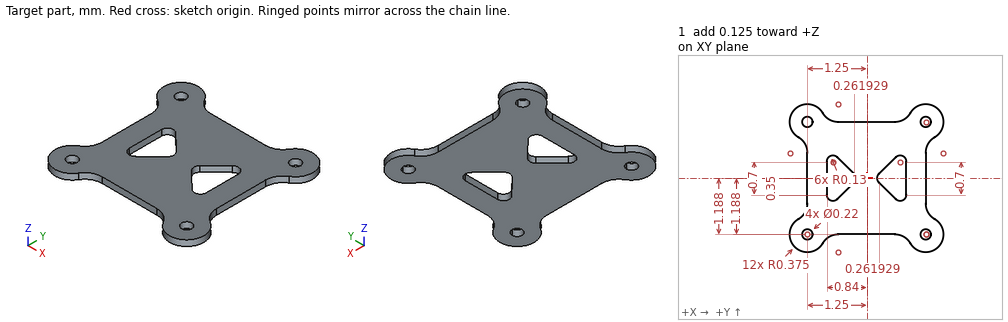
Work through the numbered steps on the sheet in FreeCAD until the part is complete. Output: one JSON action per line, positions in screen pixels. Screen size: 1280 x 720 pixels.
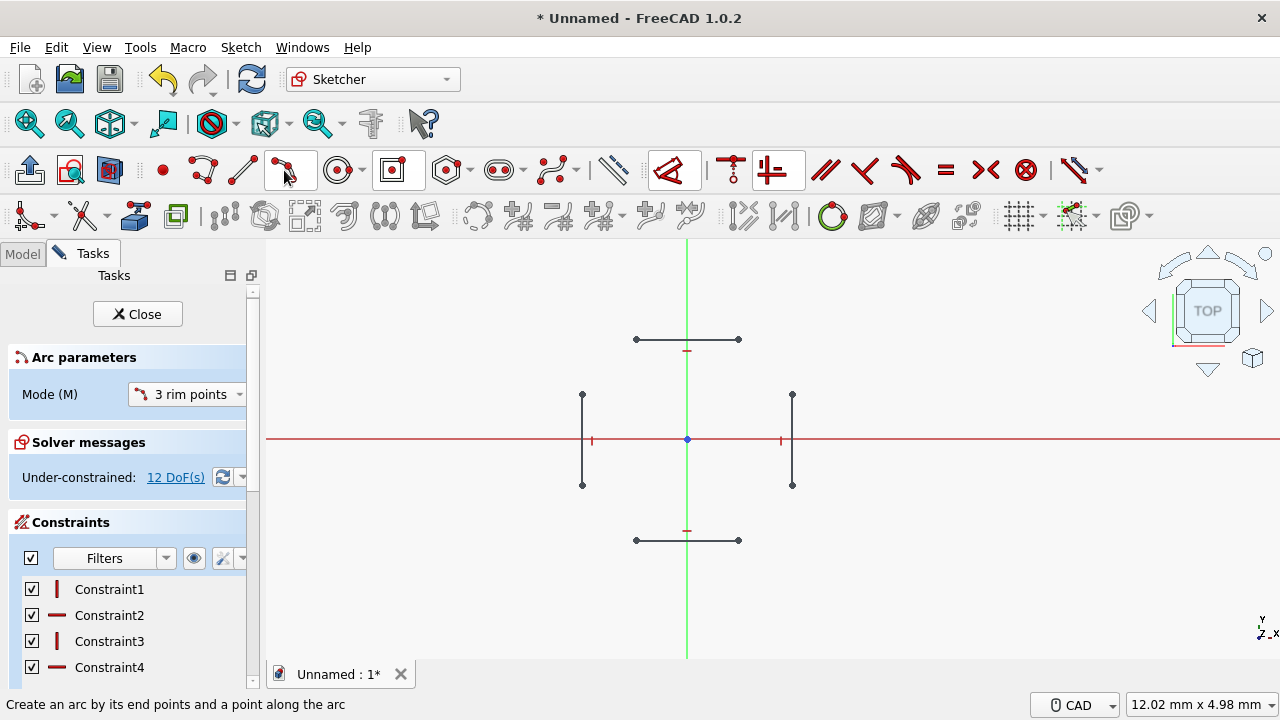
{"action": "left_click", "coordinate": [582, 486]}
{"action": "left_click", "coordinate": [566, 512]}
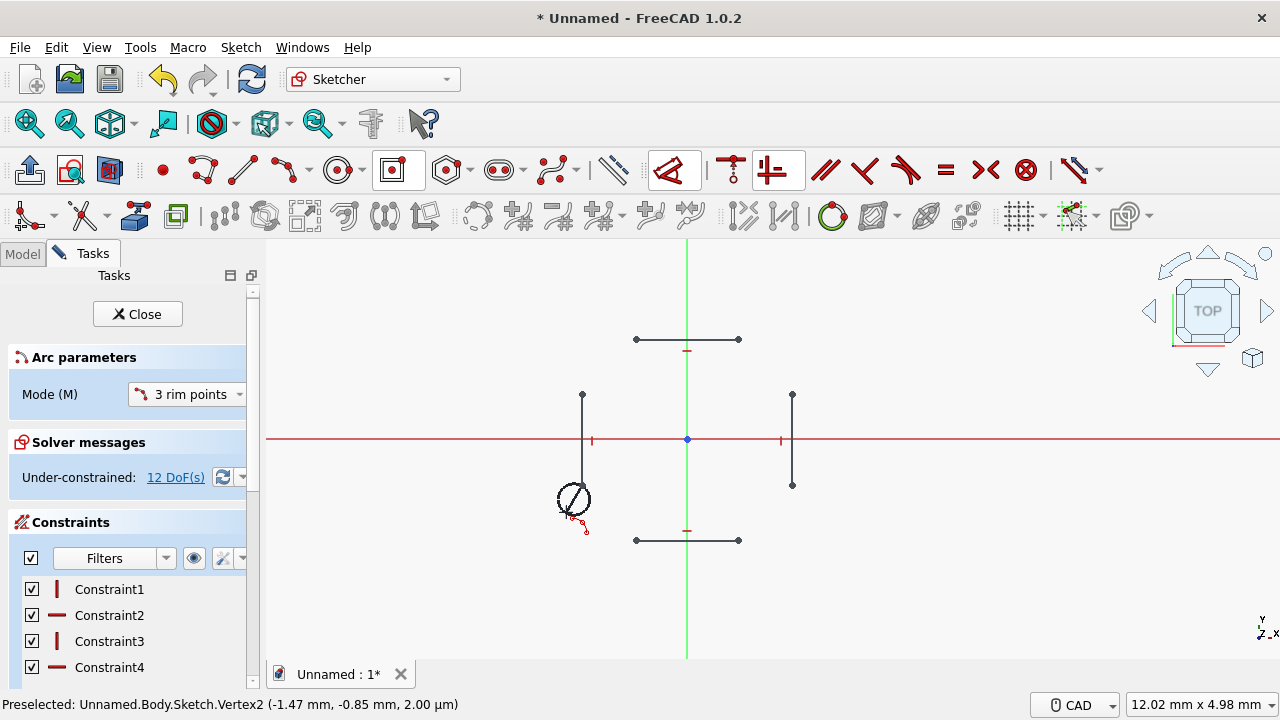
{"action": "scroll", "coordinate": [577, 501], "scroll_direction": "up", "scroll_amount": 7}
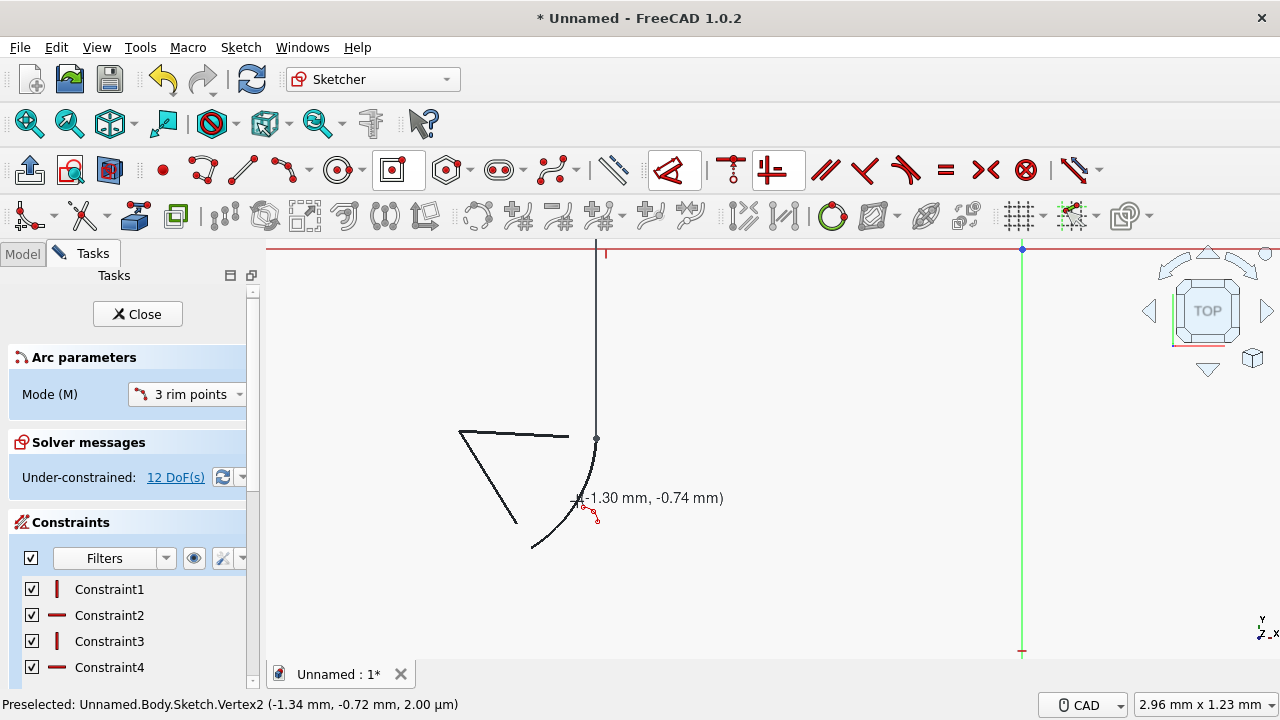
{"action": "left_click", "coordinate": [577, 498]}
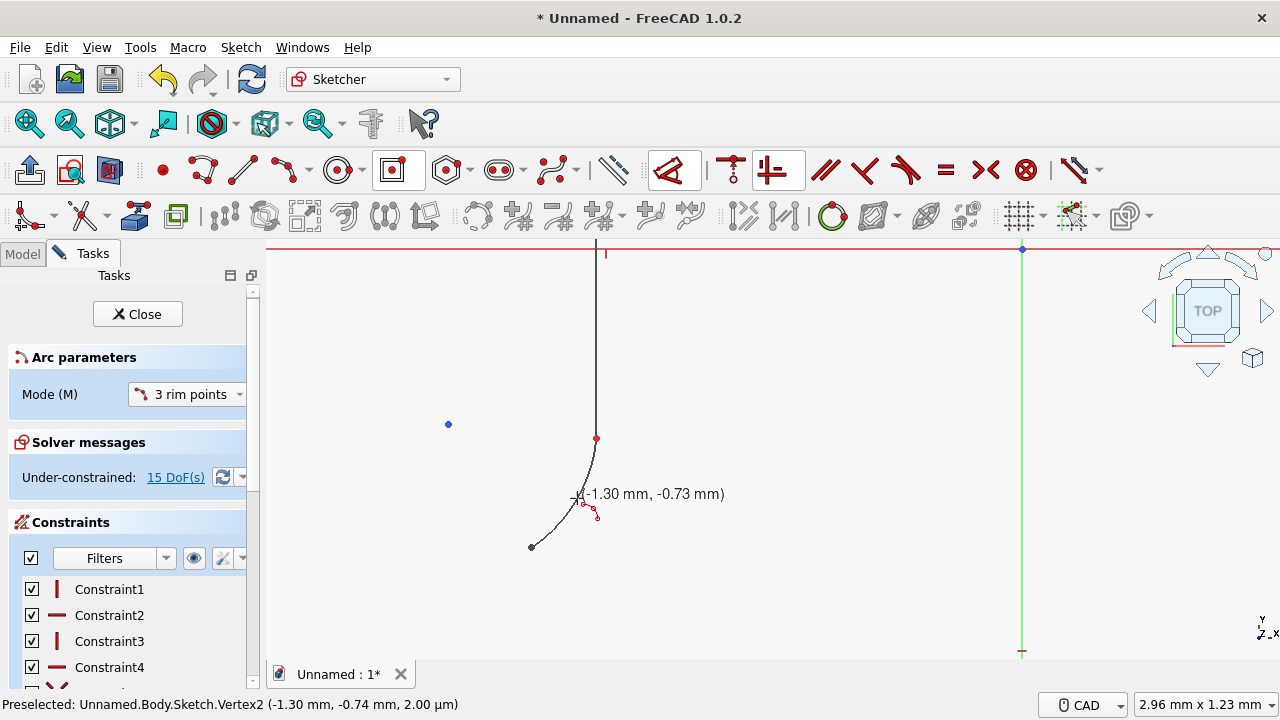
{"action": "scroll", "coordinate": [600, 514], "scroll_direction": "down", "scroll_amount": 7}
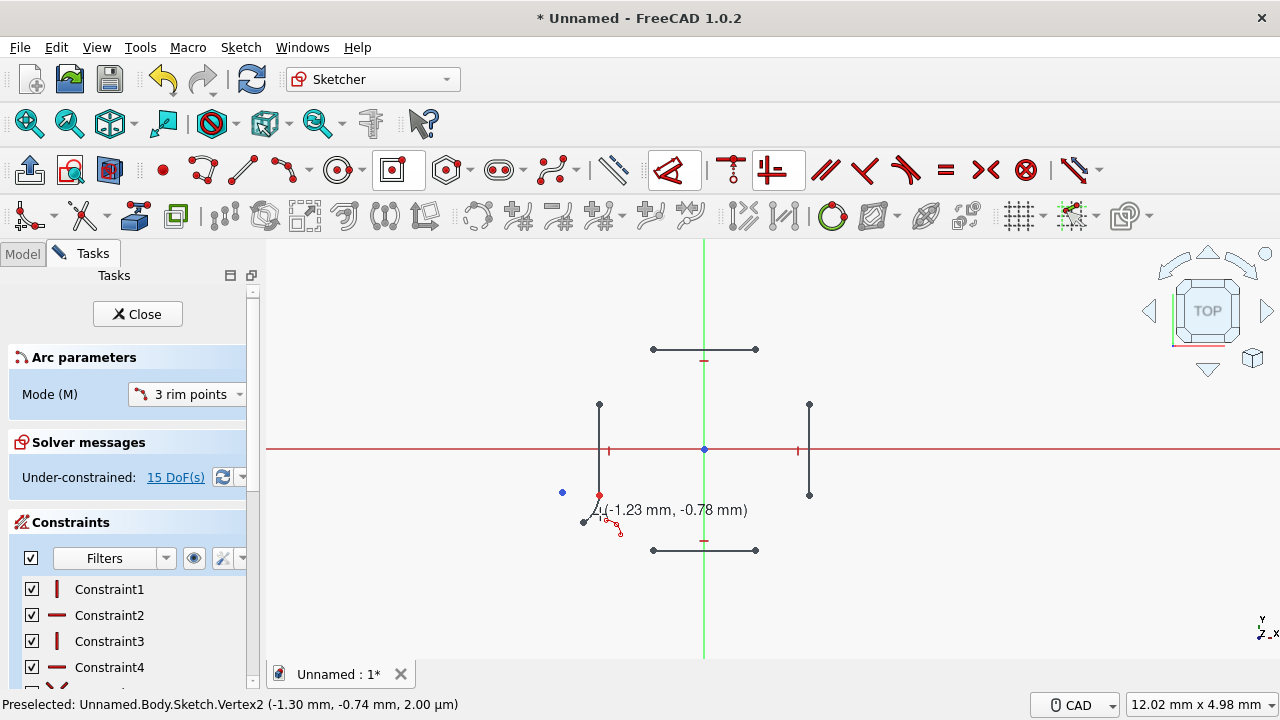
{"action": "left_click", "coordinate": [583, 523]}
{"action": "left_click", "coordinate": [626, 565]}
{"action": "left_click", "coordinate": [577, 572]}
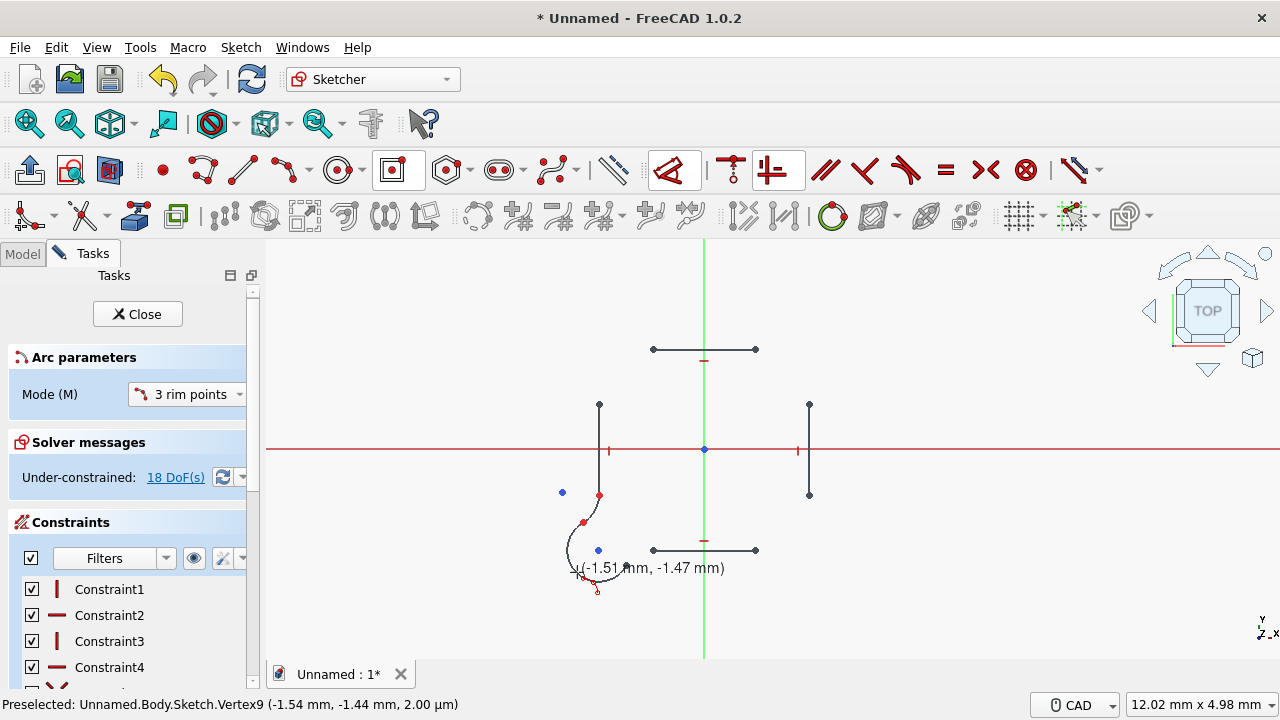
{"action": "left_click", "coordinate": [626, 566]}
{"action": "left_click", "coordinate": [653, 551]}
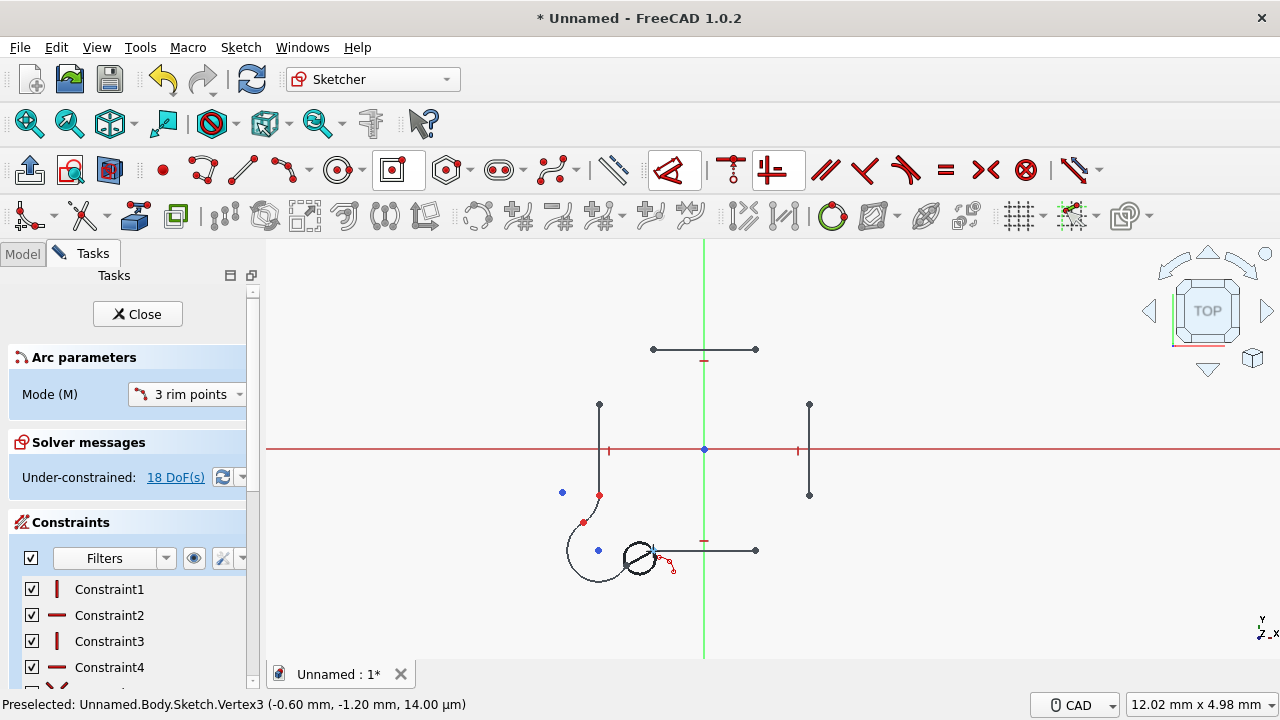
{"action": "scroll", "coordinate": [638, 554], "scroll_direction": "up", "scroll_amount": 7}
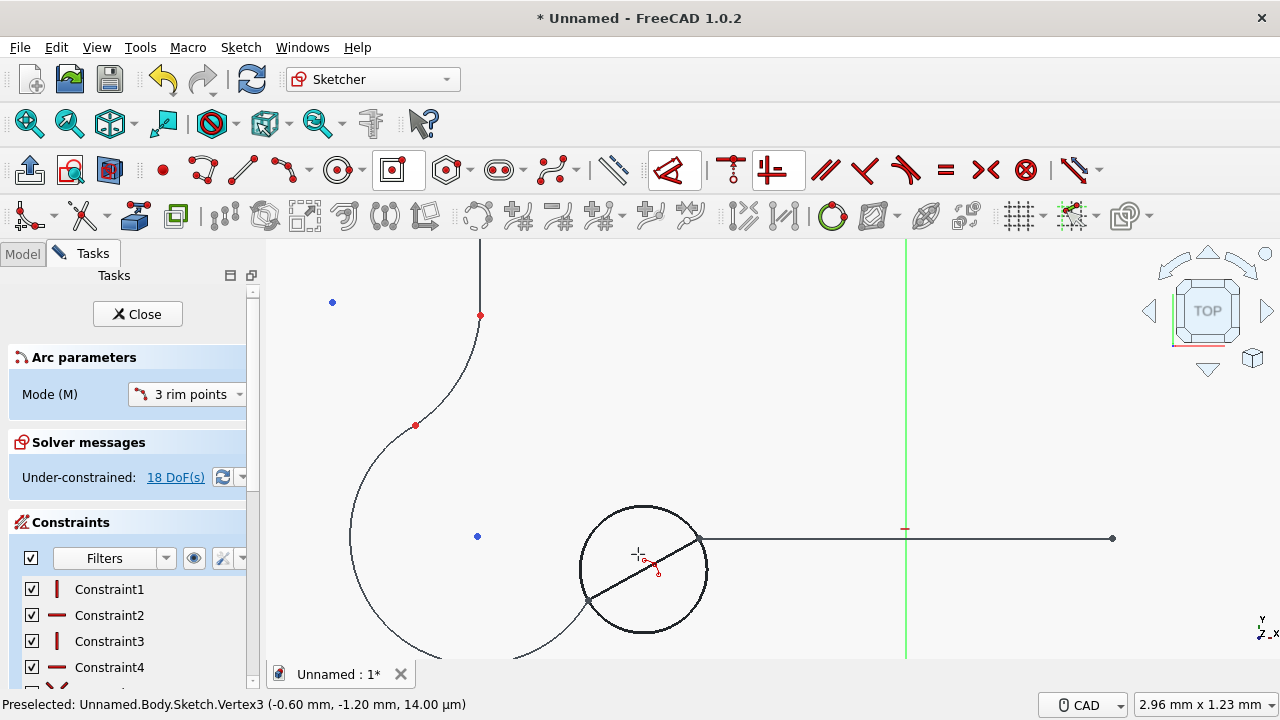
{"action": "left_click", "coordinate": [636, 551]}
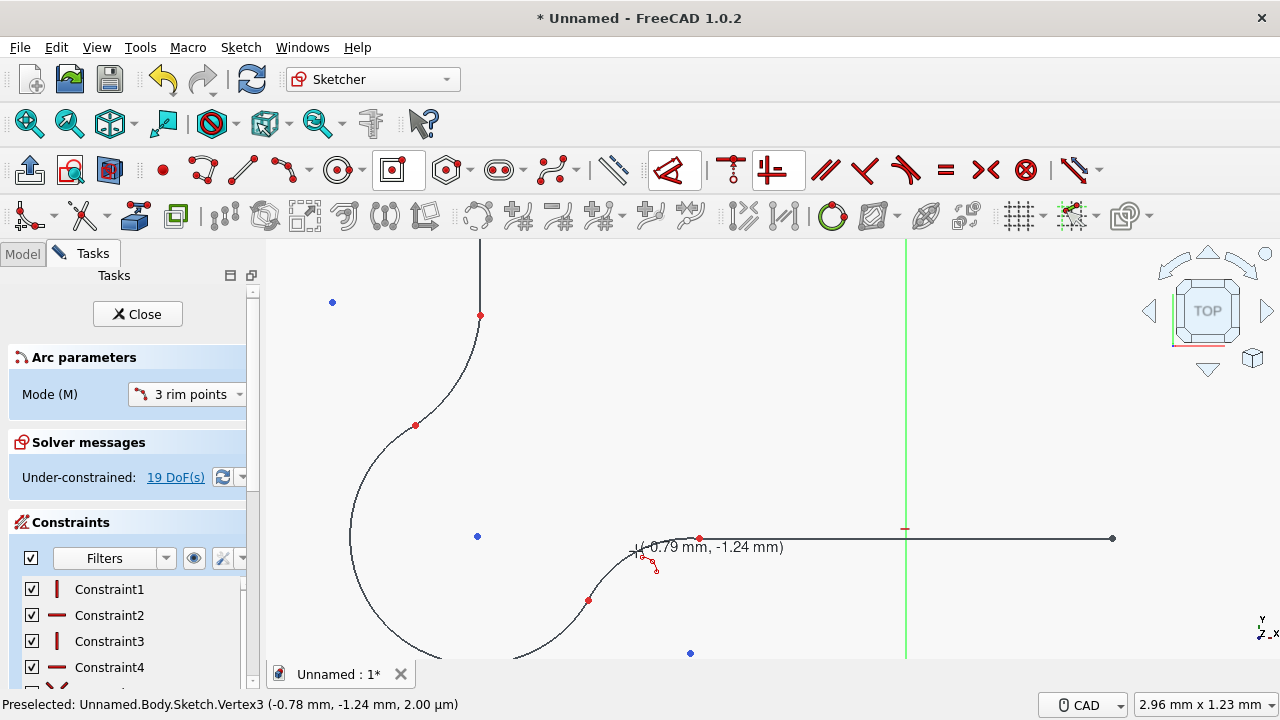
{"action": "scroll", "coordinate": [639, 554], "scroll_direction": "down", "scroll_amount": 7}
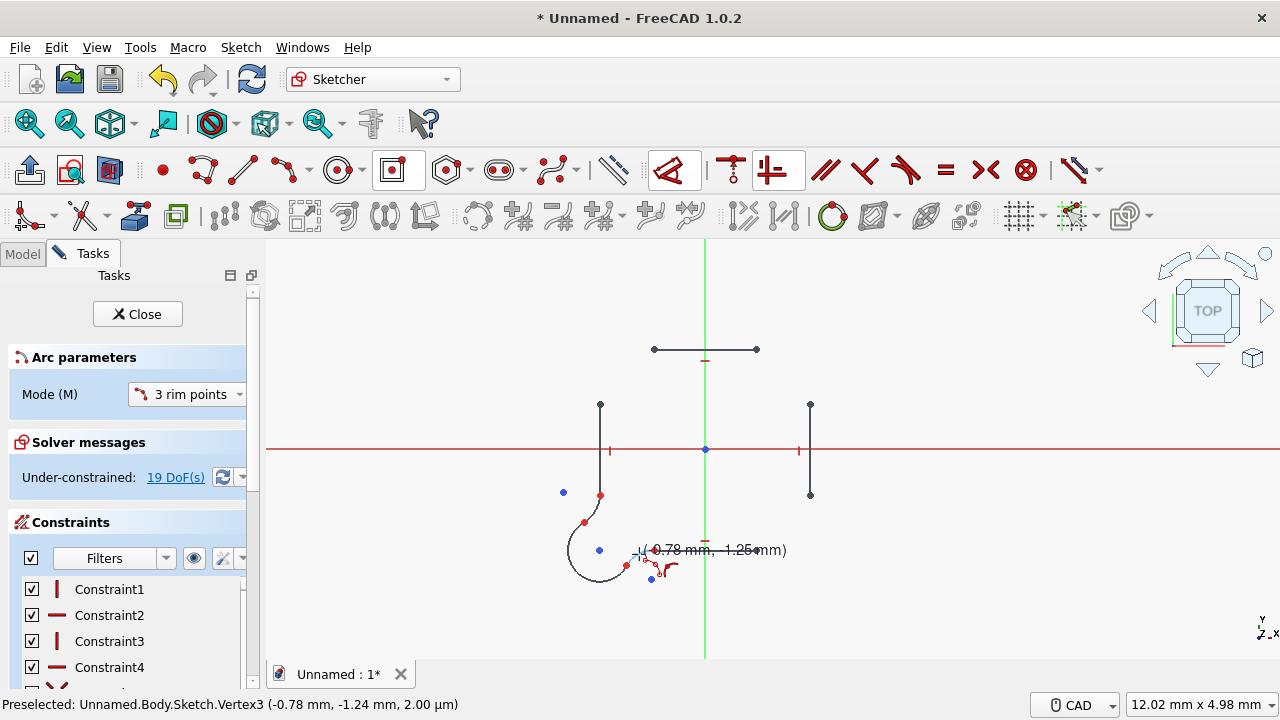
{"action": "left_click", "coordinate": [756, 551]}
{"action": "left_click", "coordinate": [783, 565]}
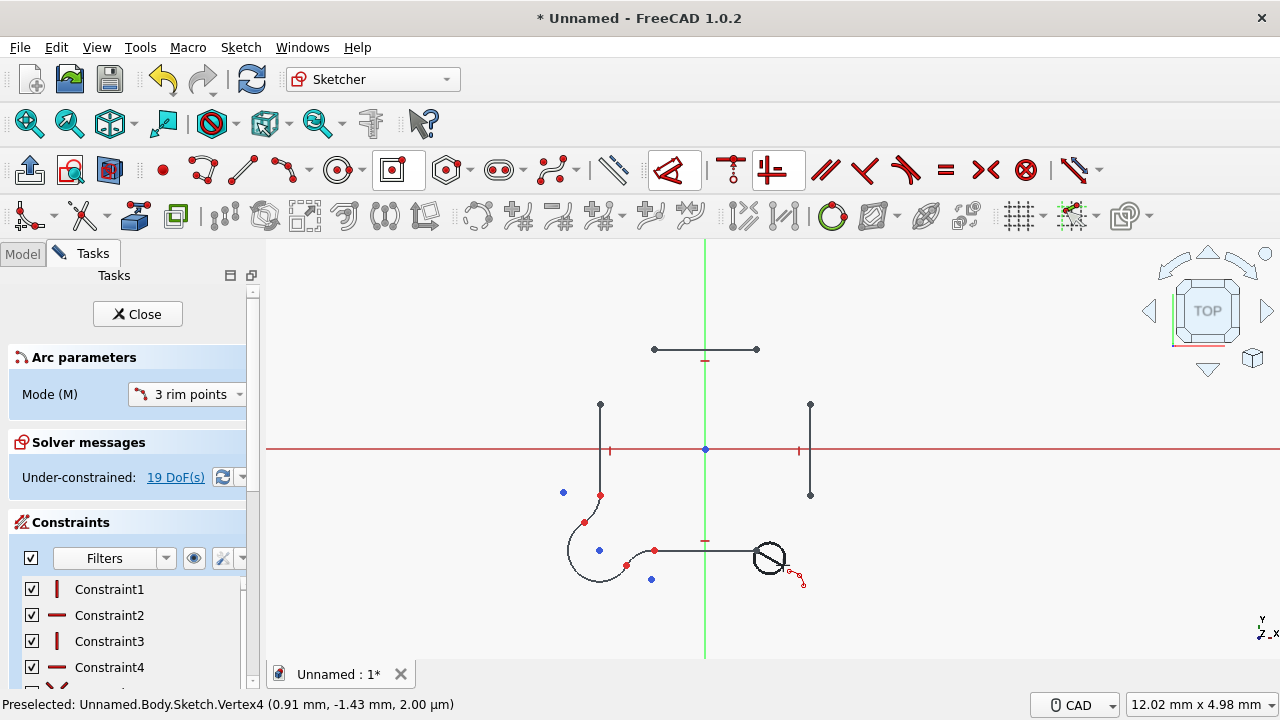
{"action": "scroll", "coordinate": [772, 554], "scroll_direction": "up", "scroll_amount": 7}